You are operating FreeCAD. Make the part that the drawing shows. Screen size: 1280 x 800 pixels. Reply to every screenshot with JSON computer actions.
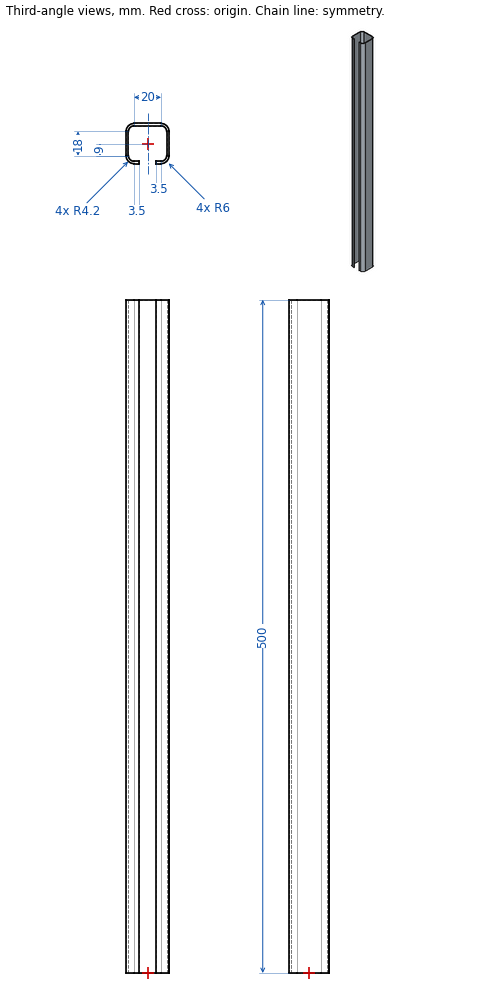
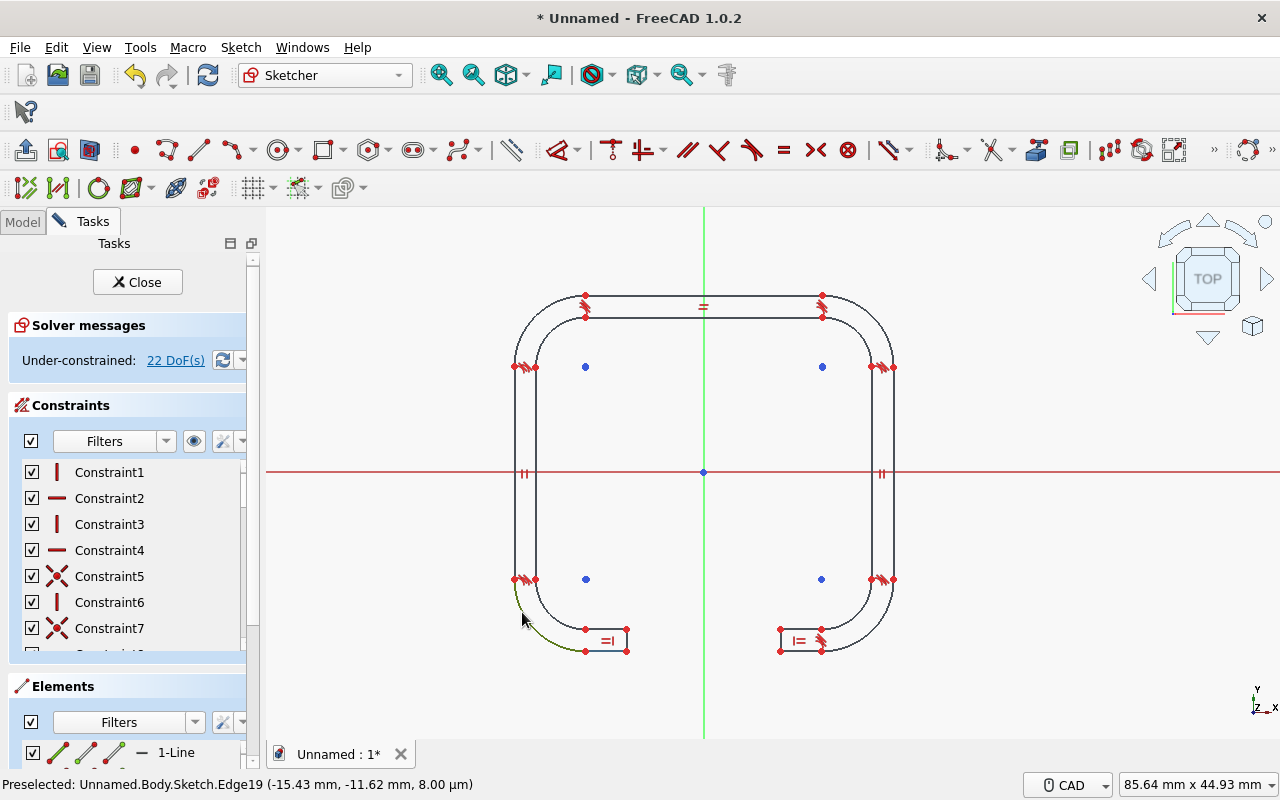
{"action": "left_click", "coordinate": [752, 150]}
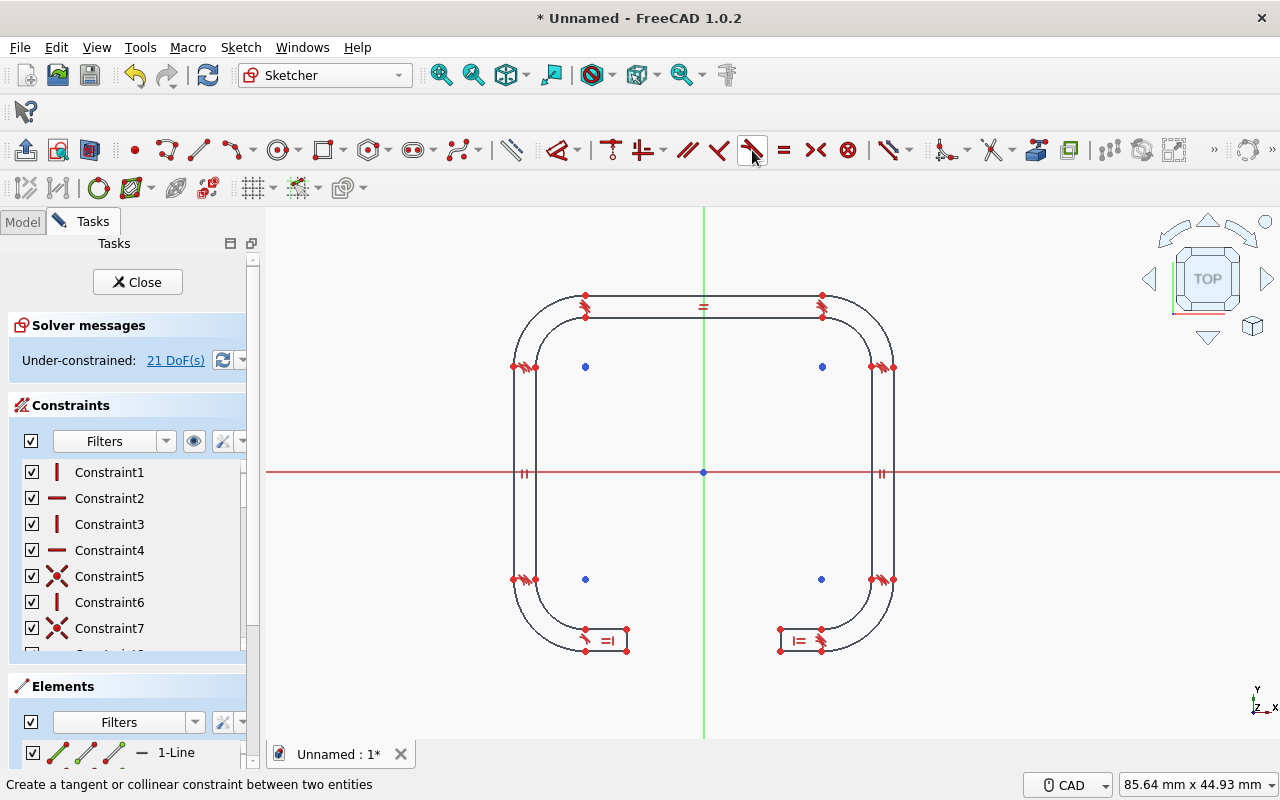
{"action": "left_click", "coordinate": [614, 629]}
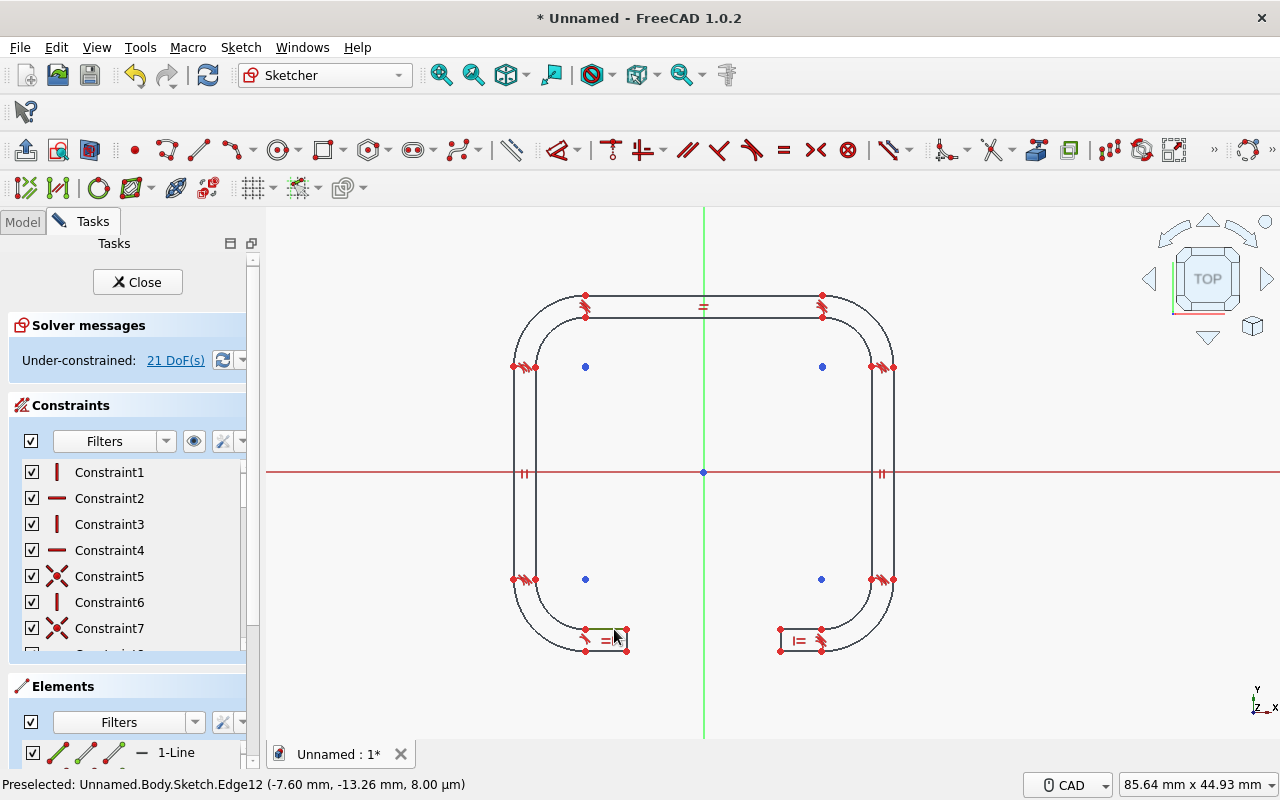
{"action": "left_click", "coordinate": [541, 602]}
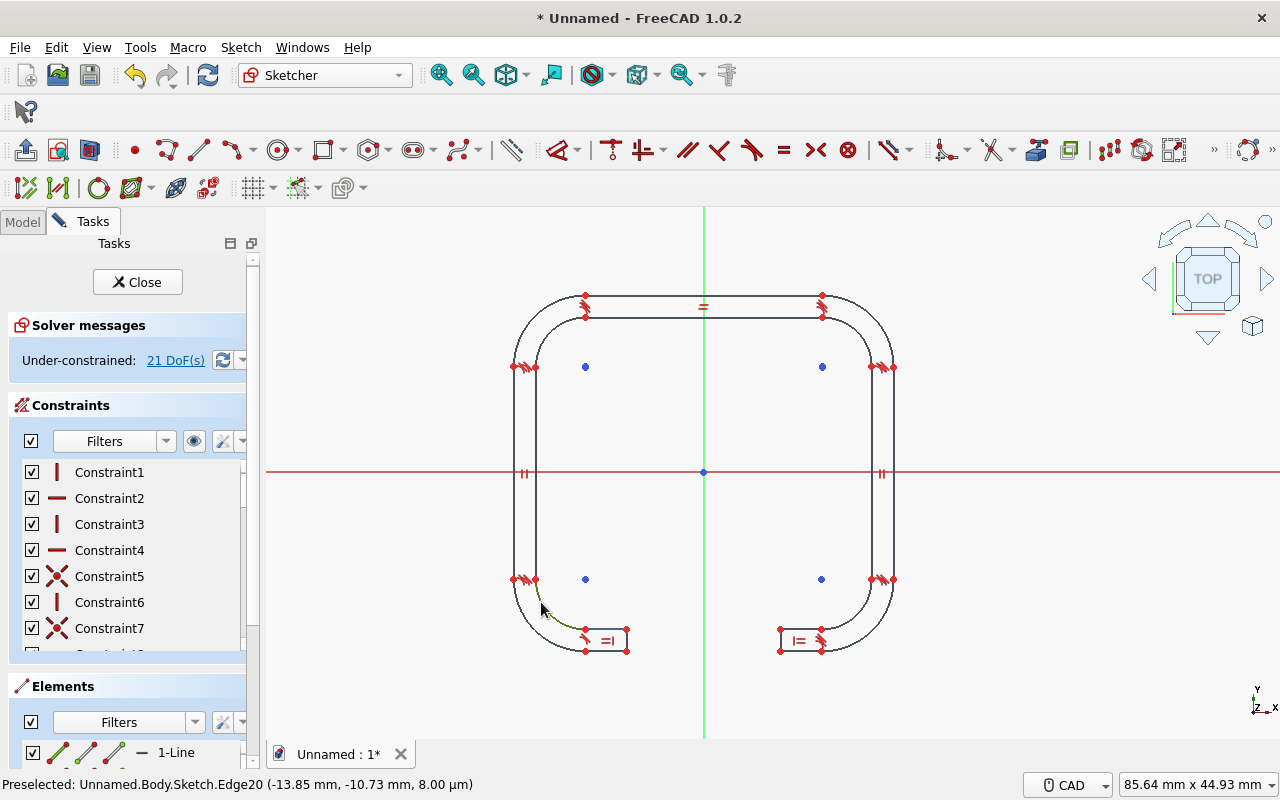
{"action": "left_click", "coordinate": [752, 150]}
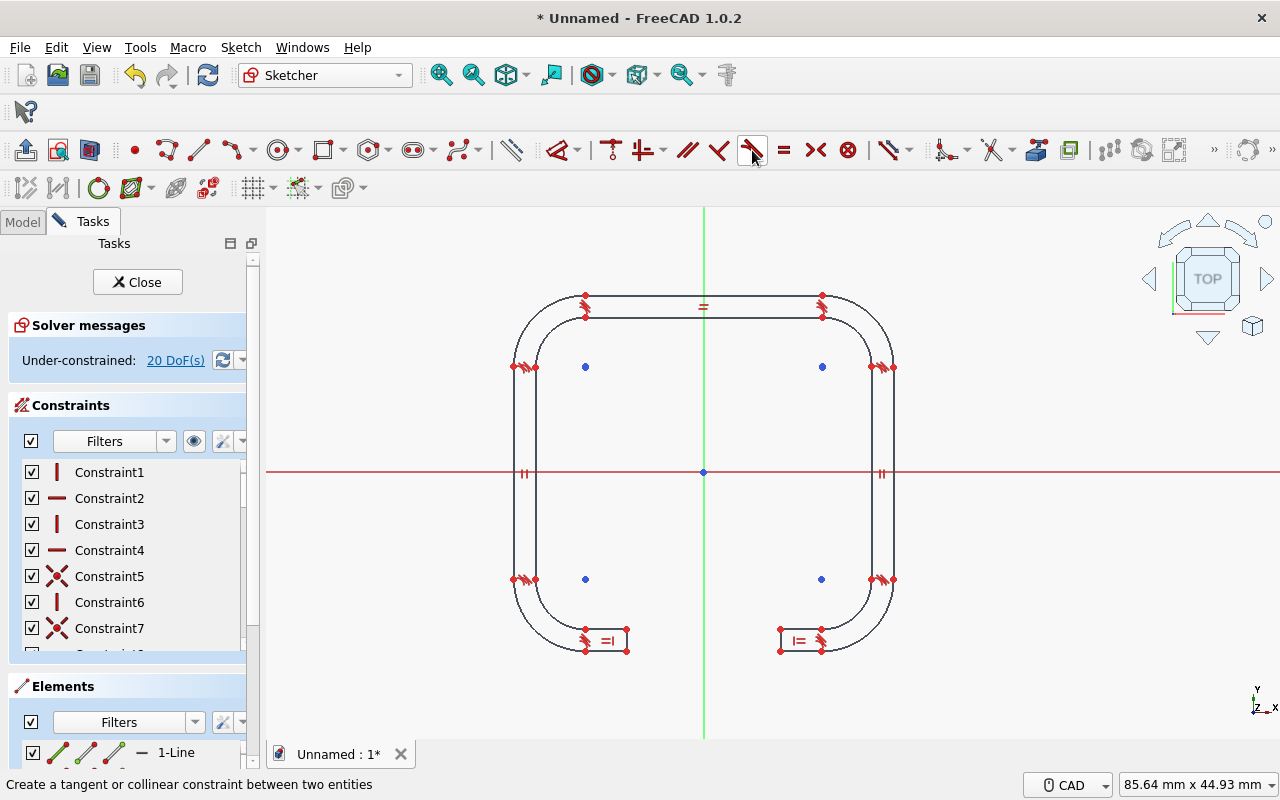
{"action": "left_click", "coordinate": [844, 624]}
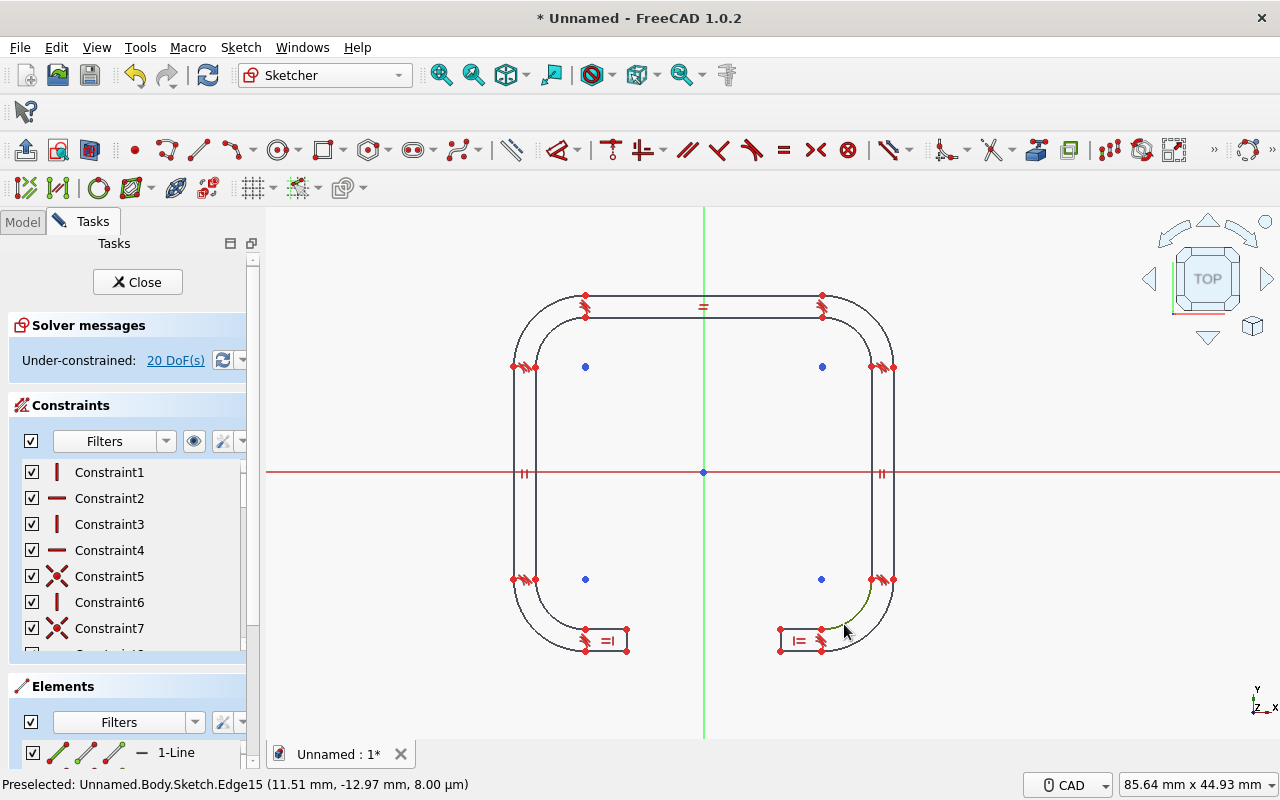
{"action": "left_click", "coordinate": [854, 644]}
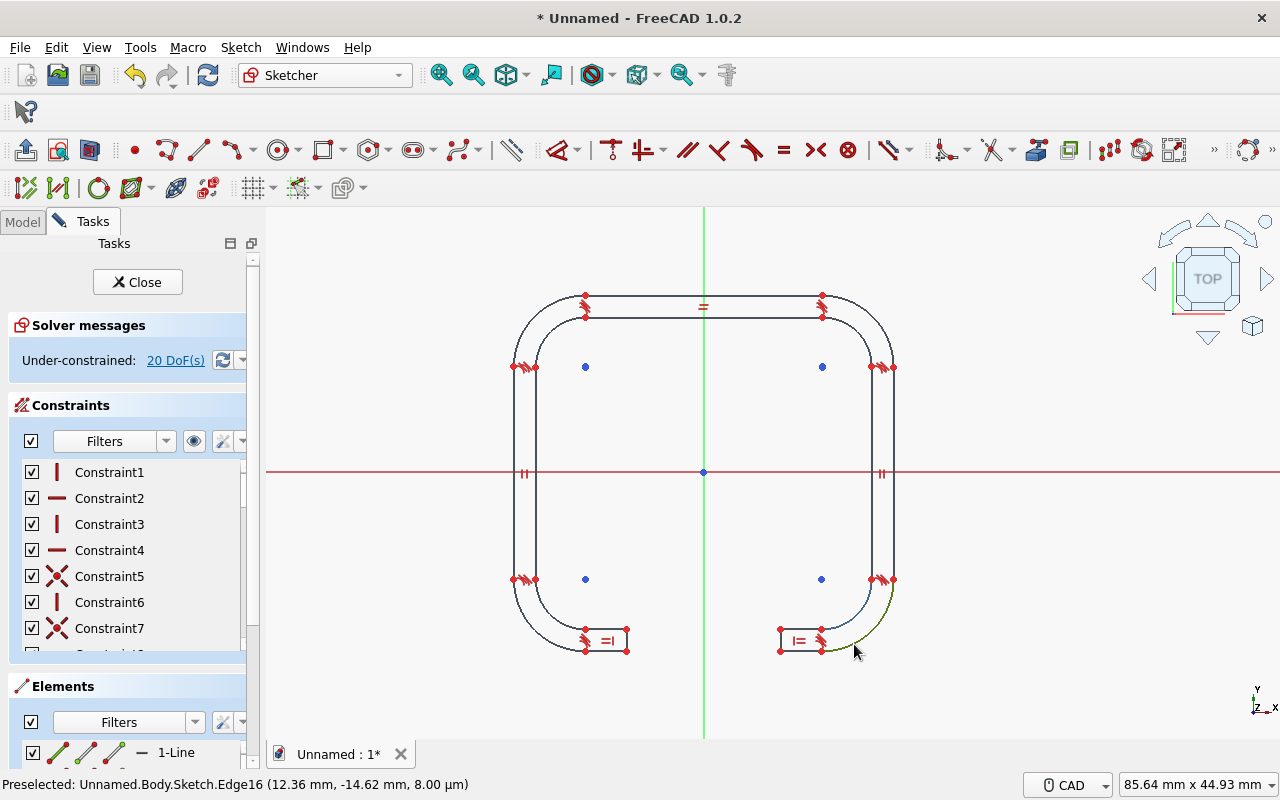
{"action": "left_click", "coordinate": [612, 150]}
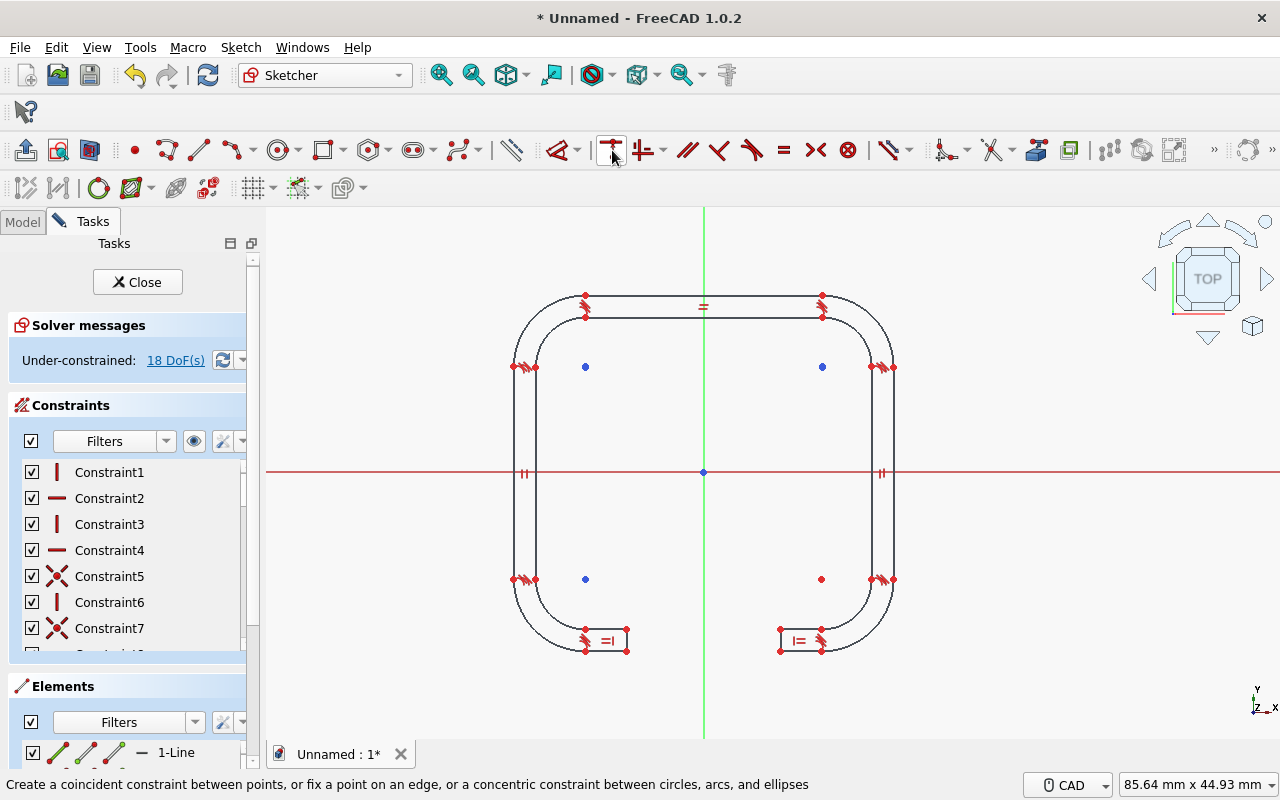
{"action": "left_click", "coordinate": [866, 344]}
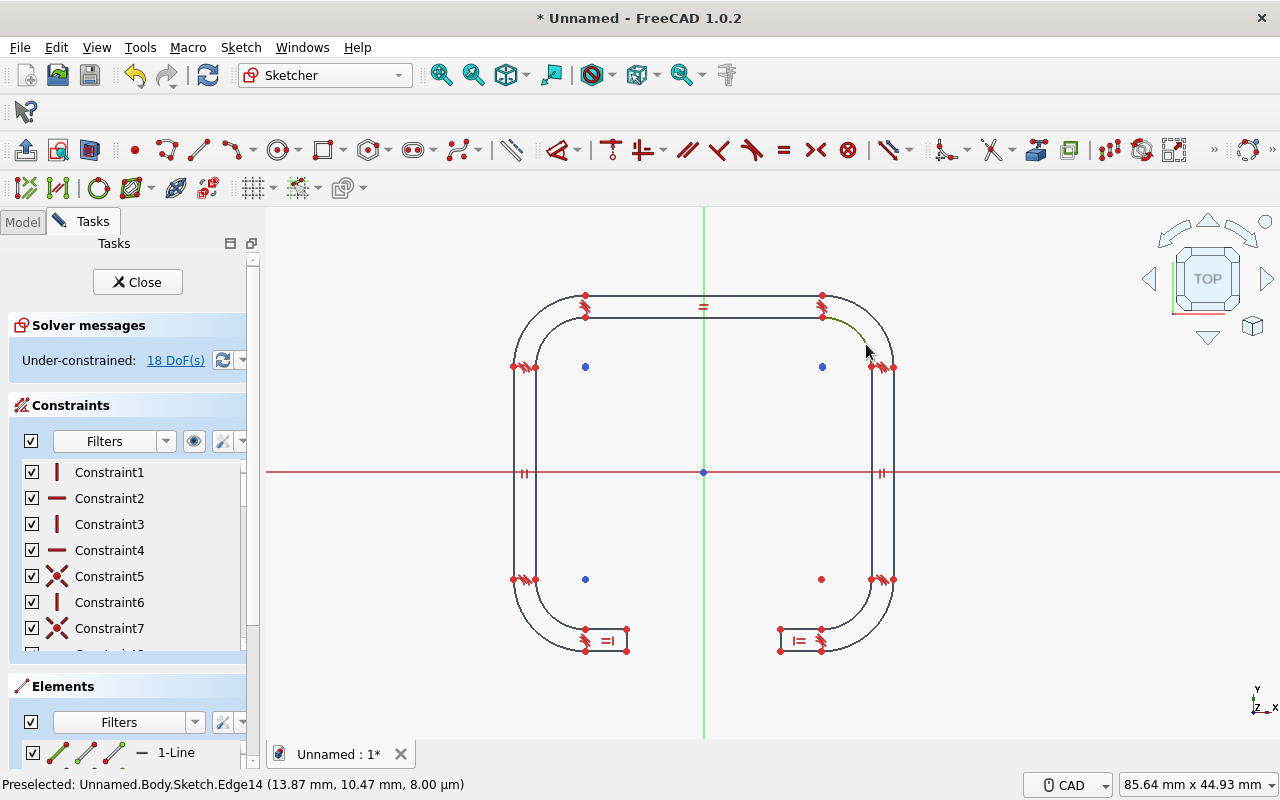
{"action": "left_click", "coordinate": [886, 335]}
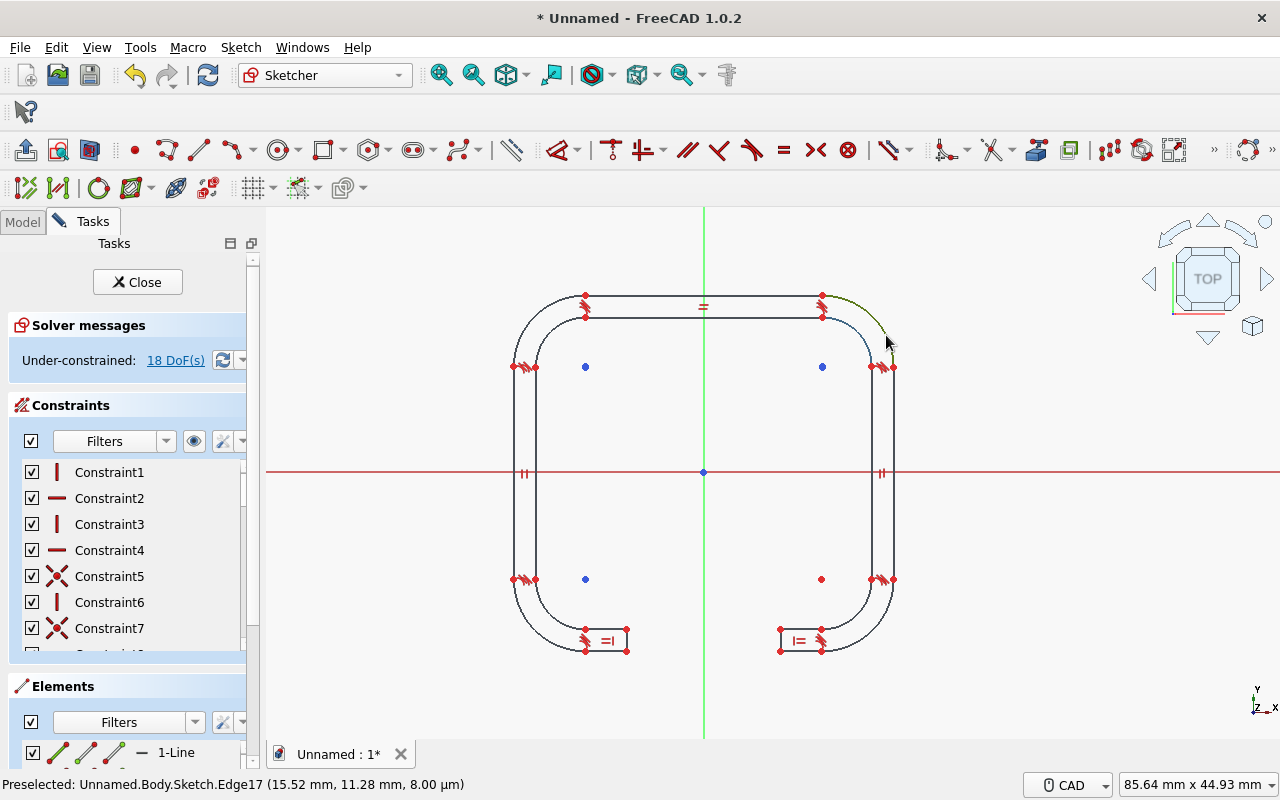
{"action": "left_click", "coordinate": [612, 150]}